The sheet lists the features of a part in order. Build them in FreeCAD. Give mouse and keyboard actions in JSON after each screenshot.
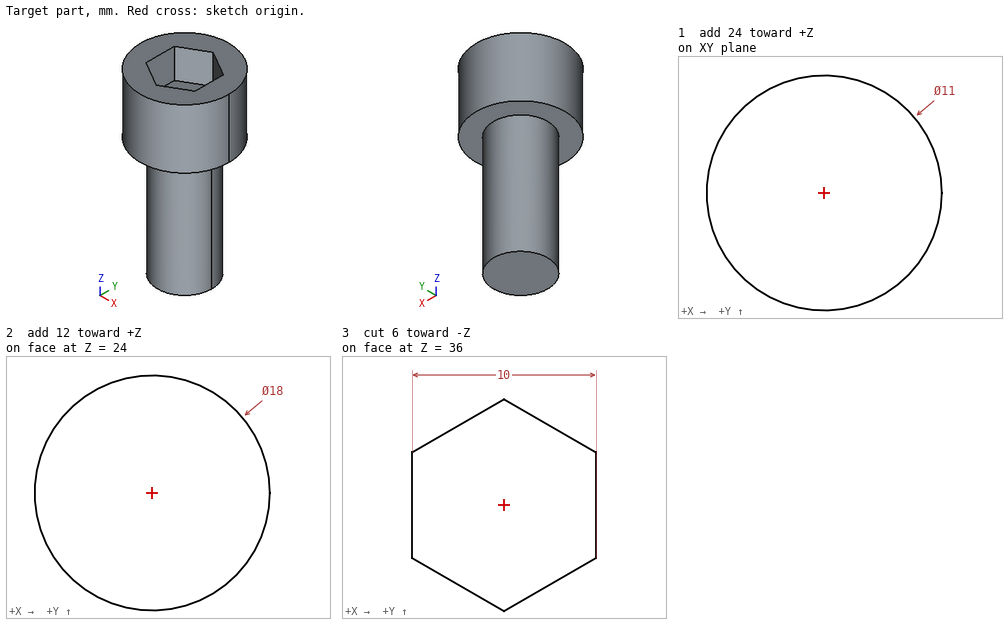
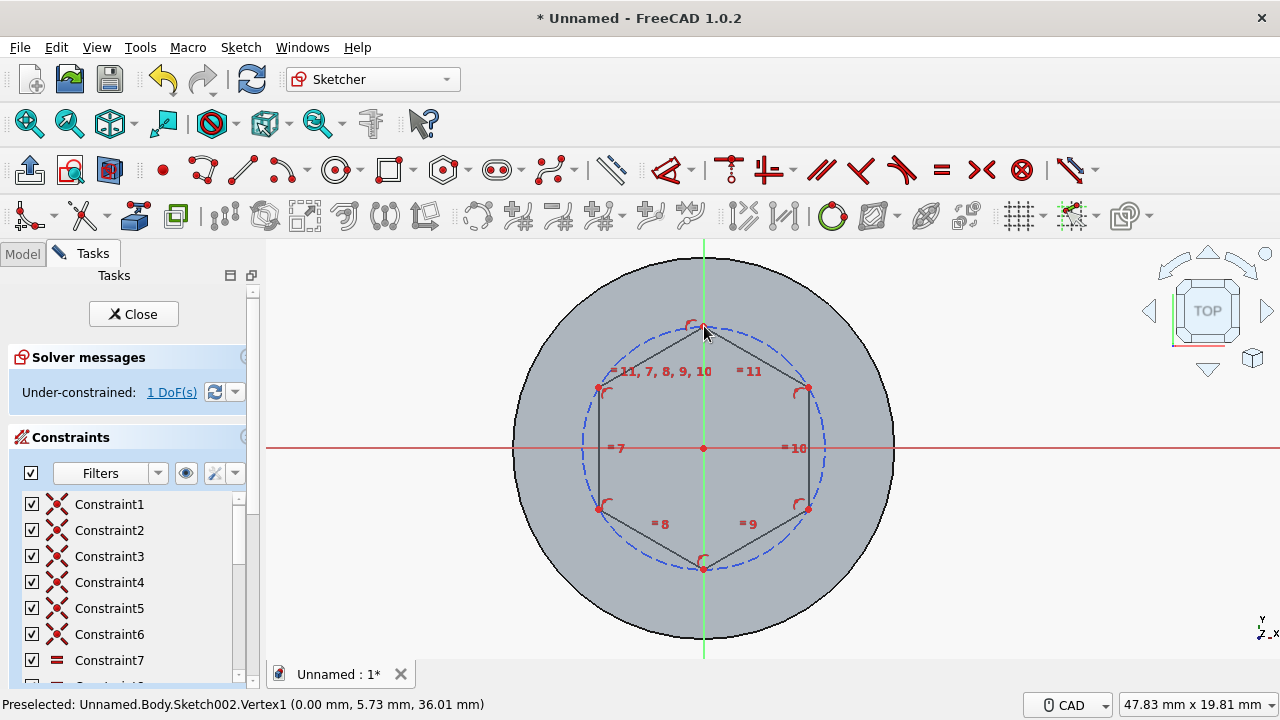
{"action": "left_click", "coordinate": [666, 170]}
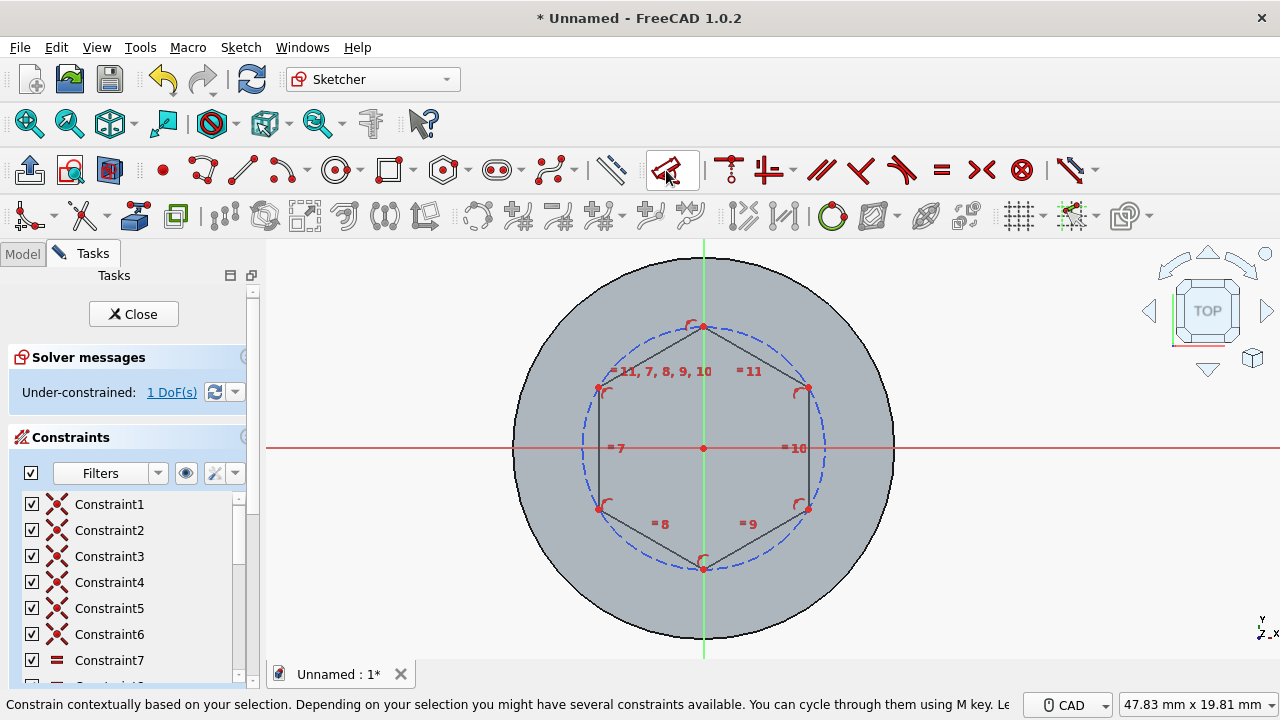
{"action": "left_click", "coordinate": [599, 388]}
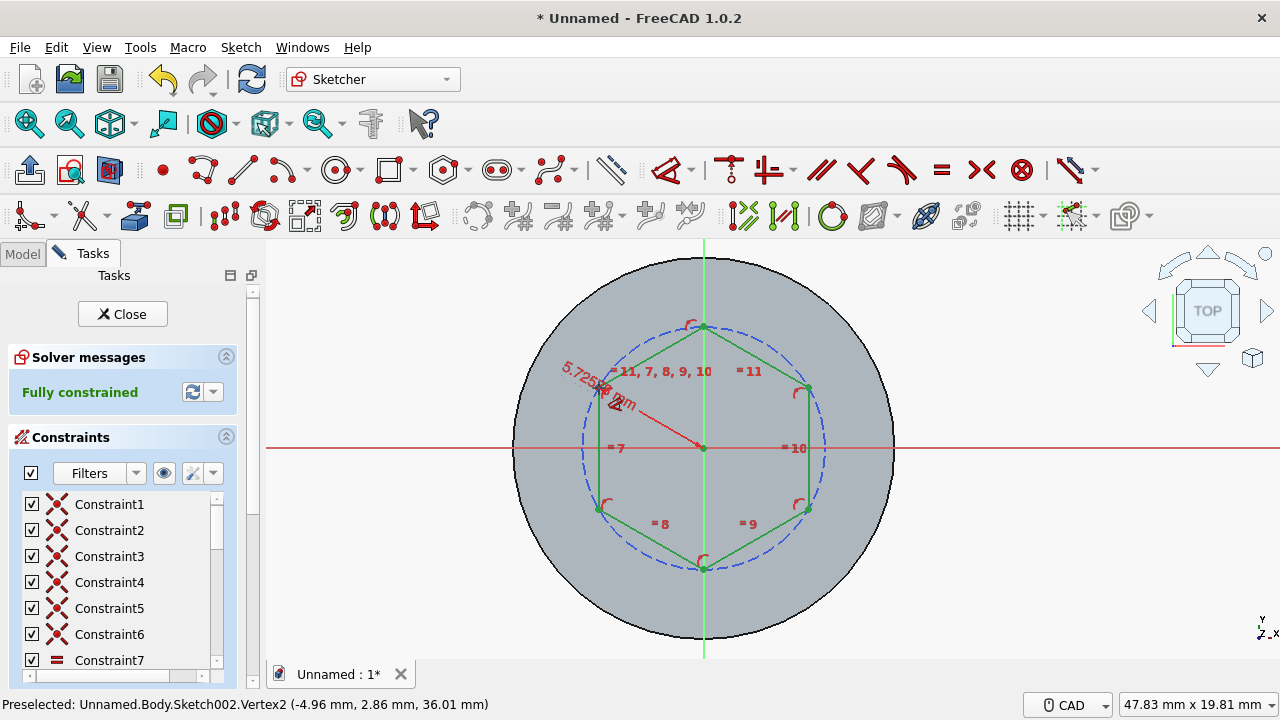
{"action": "left_click", "coordinate": [809, 509]}
{"action": "left_click", "coordinate": [630, 567]}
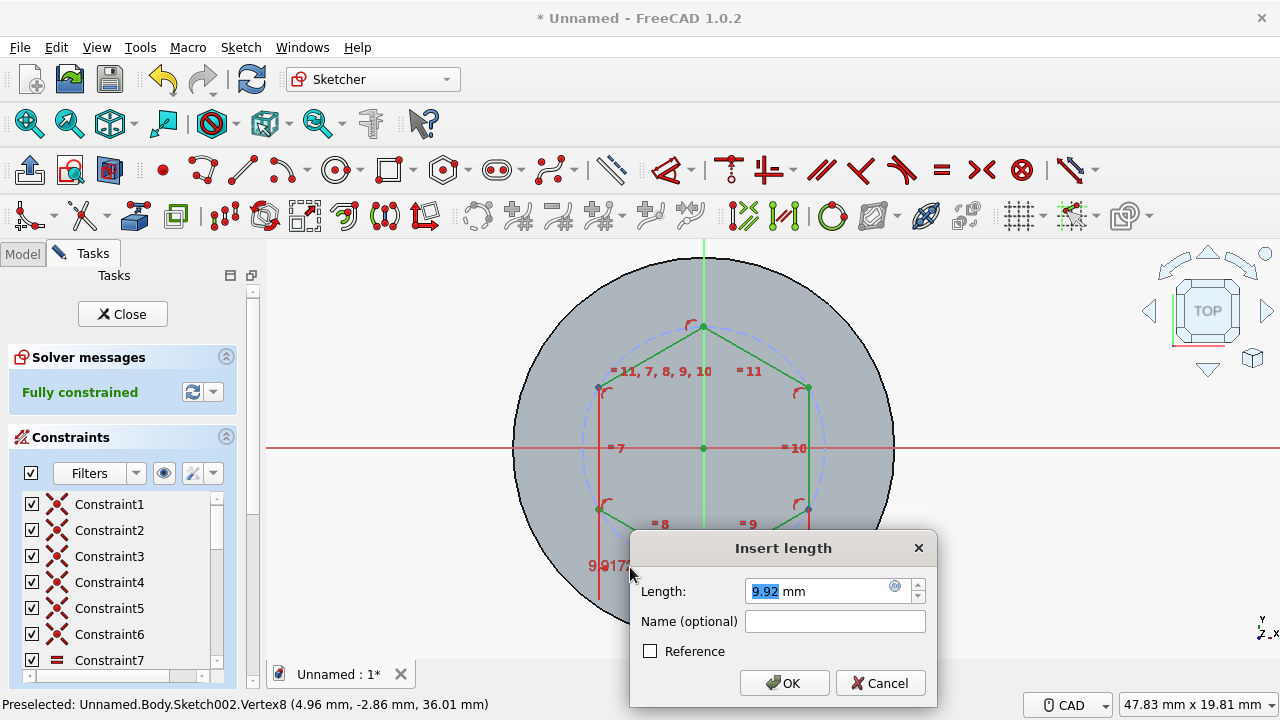
{"action": "type", "text": "10"}
{"action": "key", "text": "Return"}
{"action": "key", "text": "Escape"}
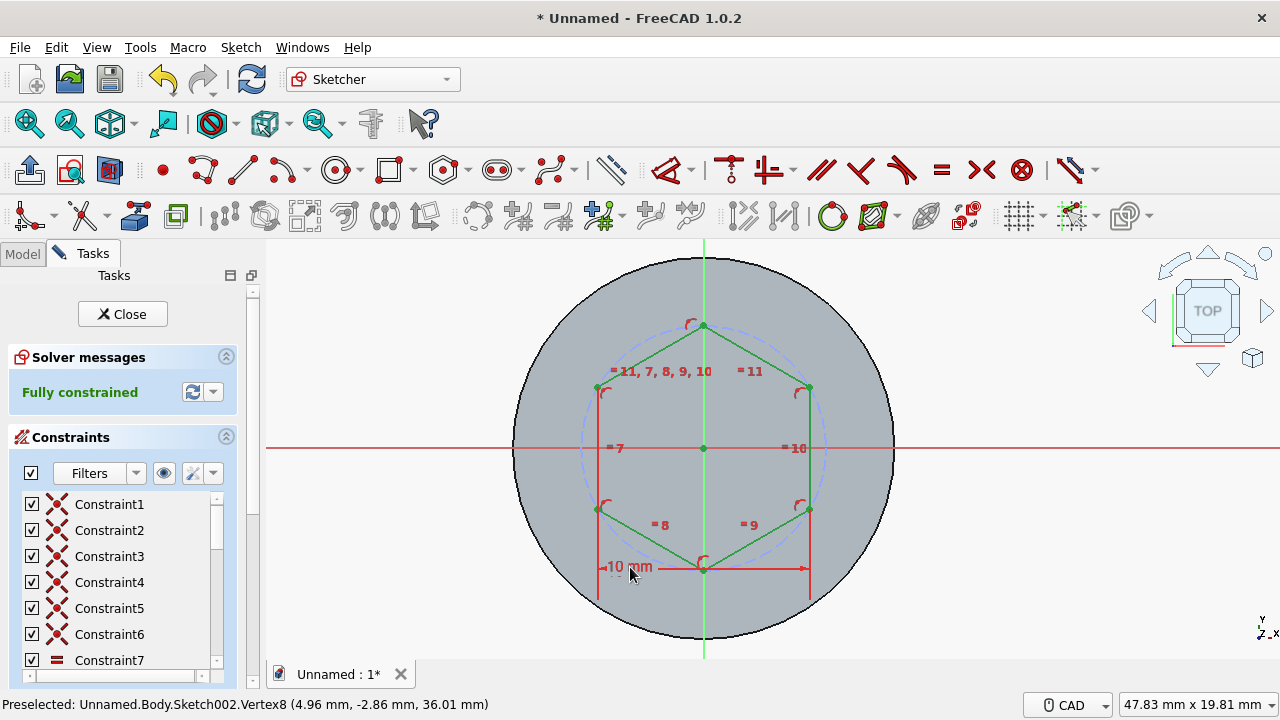
{"action": "left_click", "coordinate": [123, 314]}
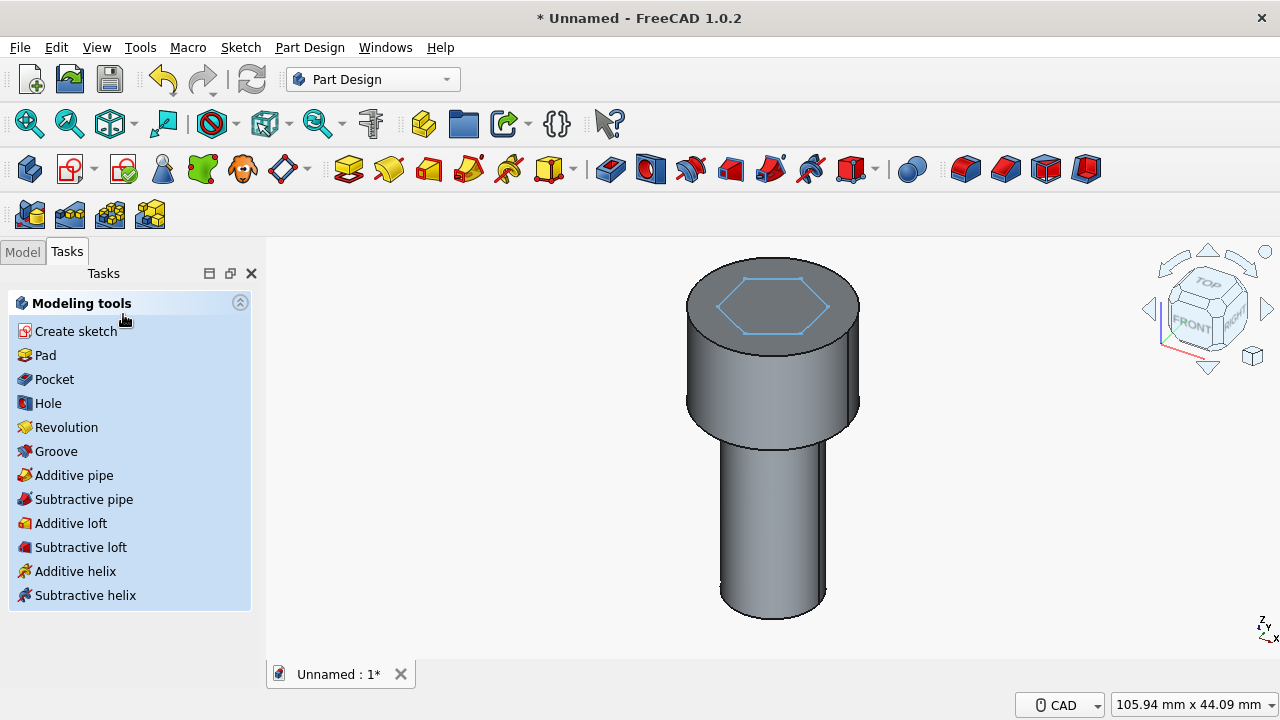
{"action": "left_click", "coordinate": [612, 170]}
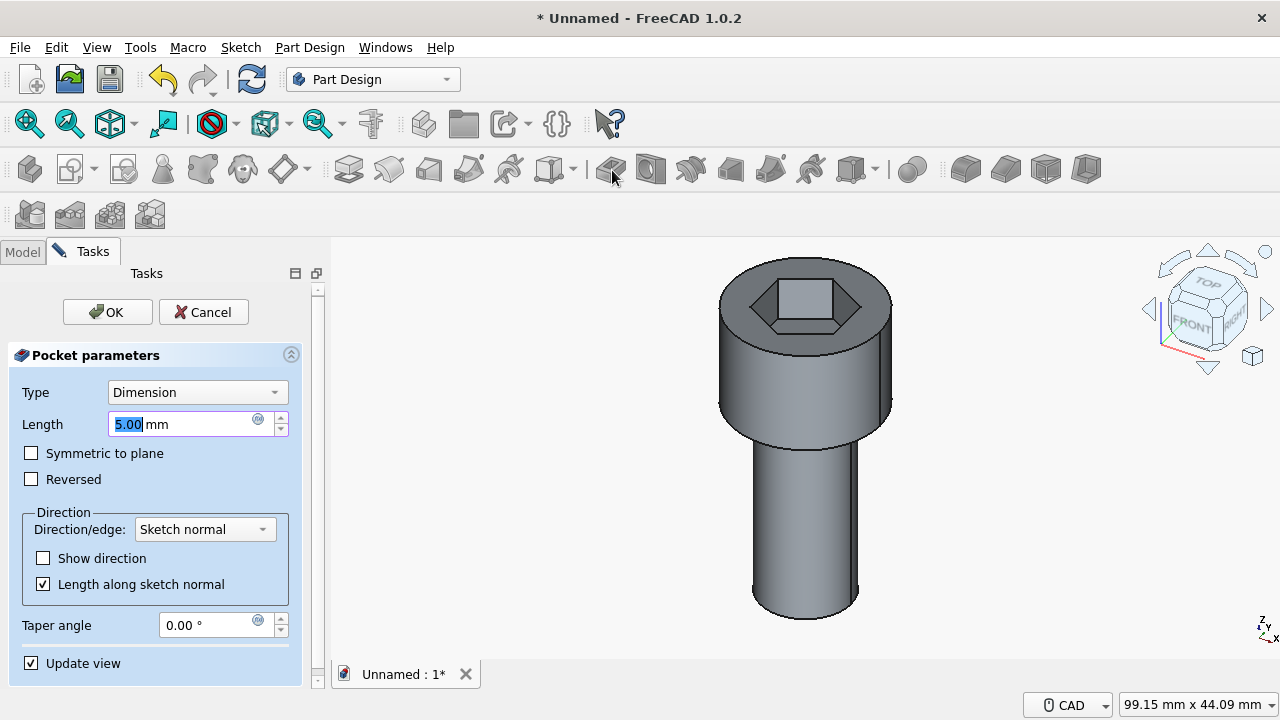
{"action": "type", "text": "6"}
{"action": "key", "text": "Tab"}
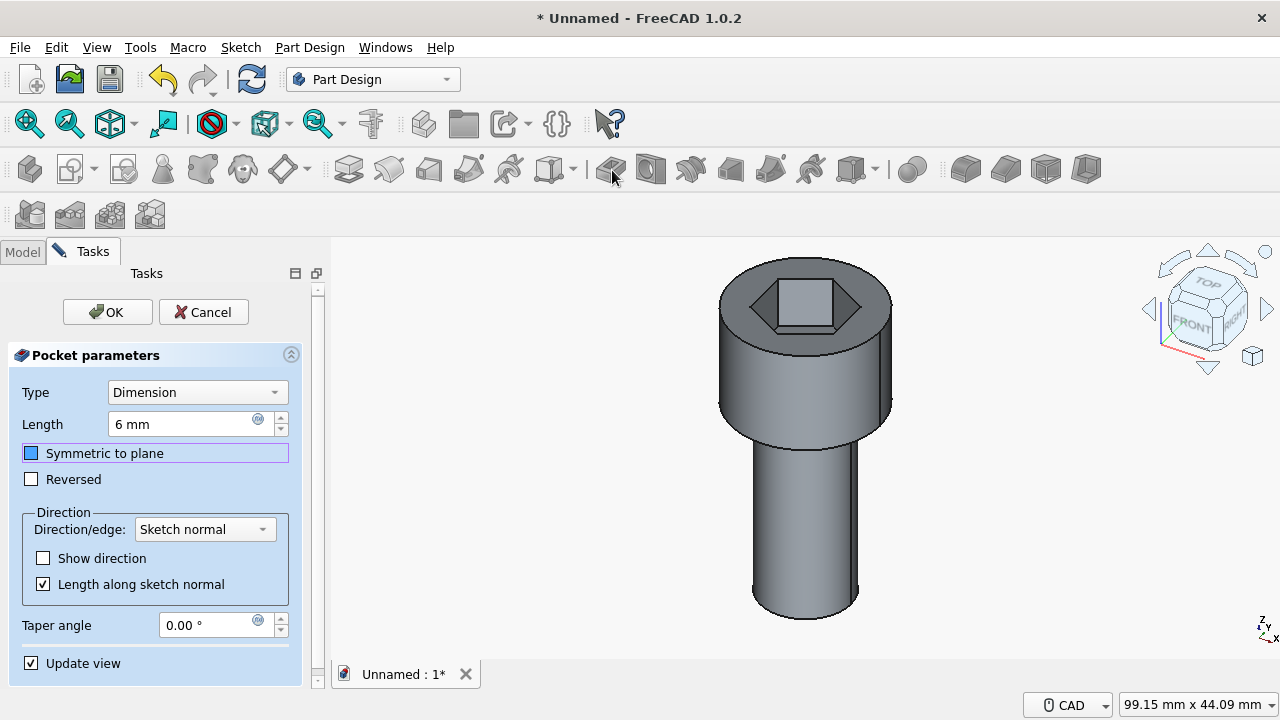
{"action": "left_click", "coordinate": [108, 312]}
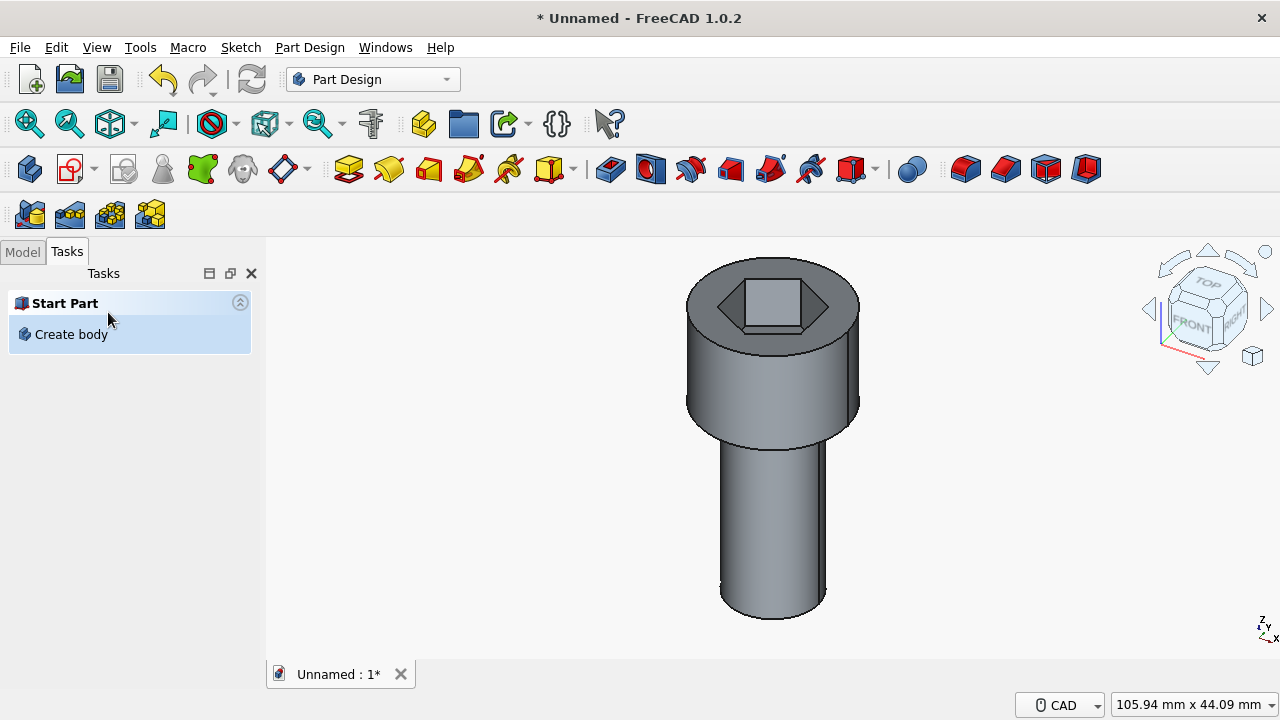
{"action": "key", "text": "0"}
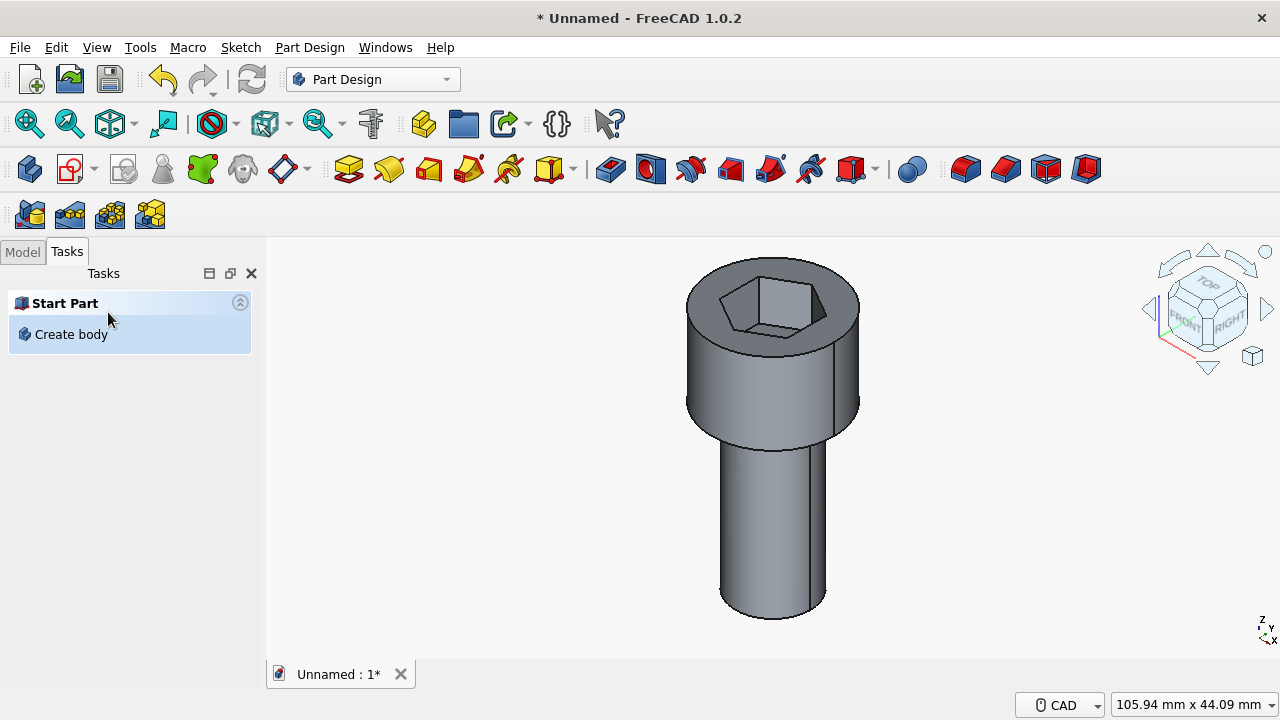
{"action": "left_click", "coordinate": [30, 124]}